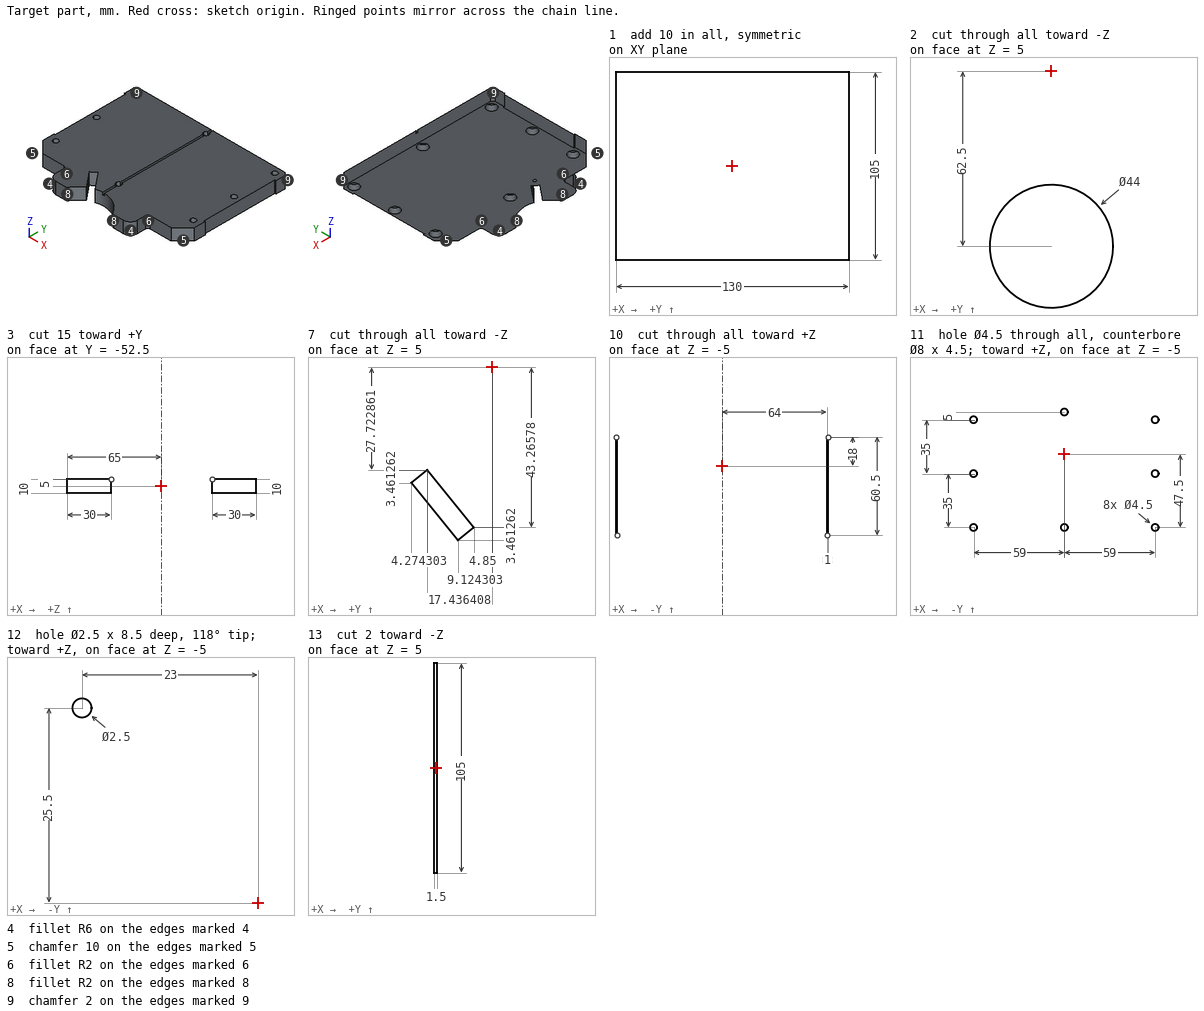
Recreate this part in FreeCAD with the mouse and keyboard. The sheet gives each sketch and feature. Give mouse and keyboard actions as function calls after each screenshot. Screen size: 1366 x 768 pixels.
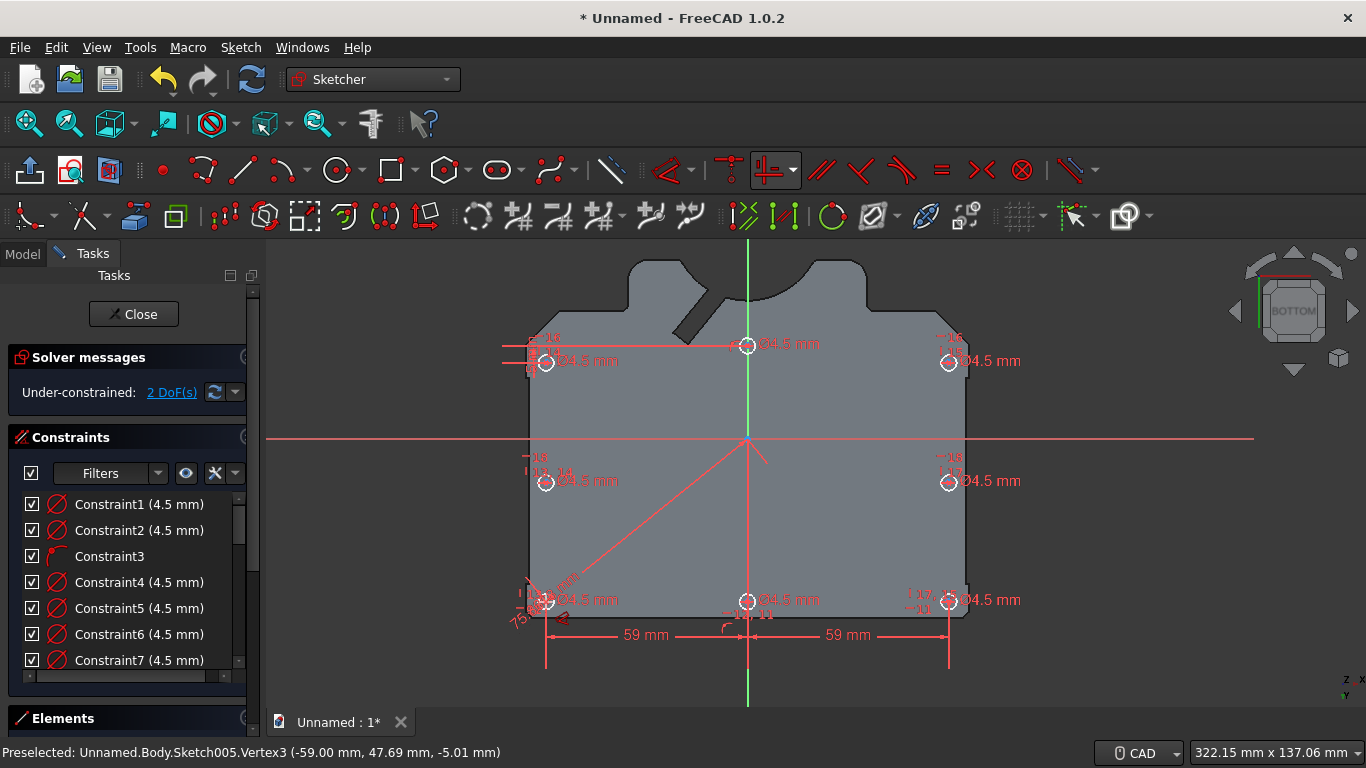
click(546, 483)
click(512, 542)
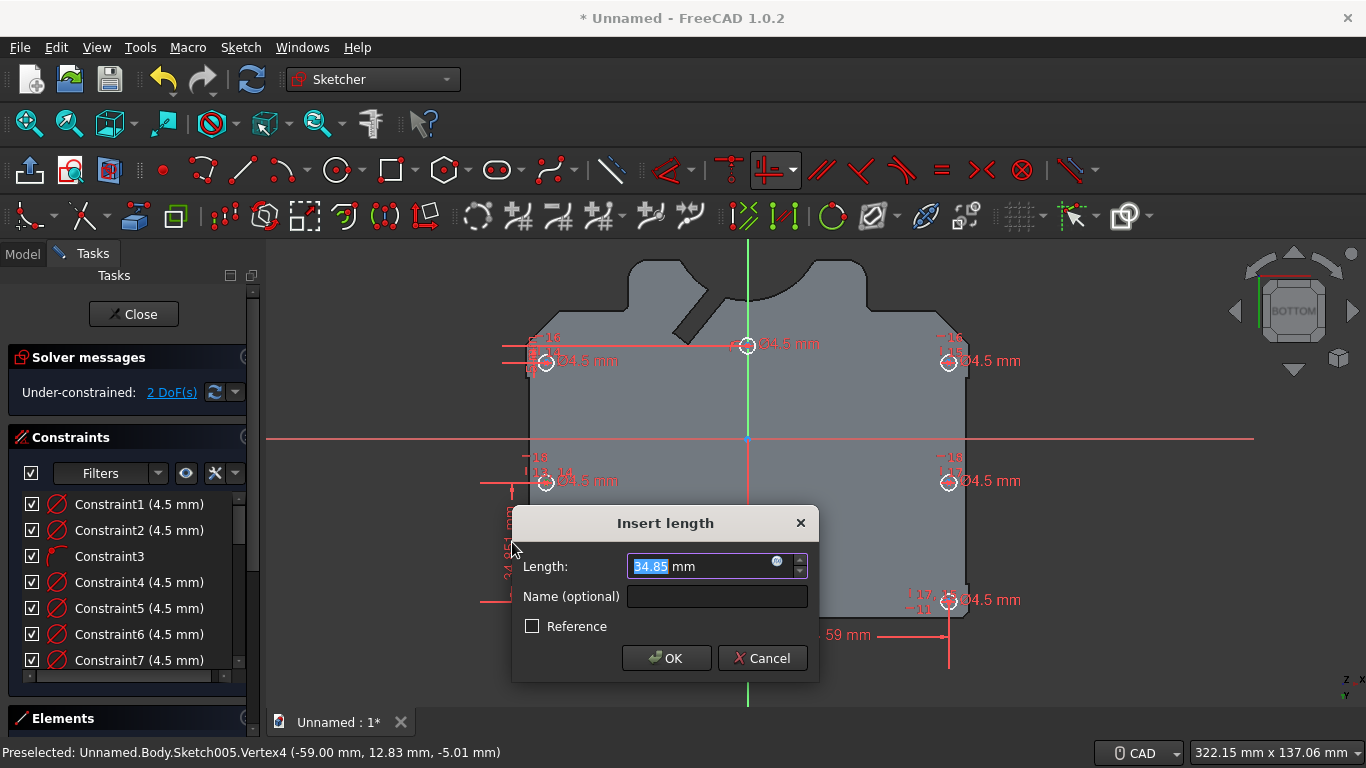
text(35)
key(Return)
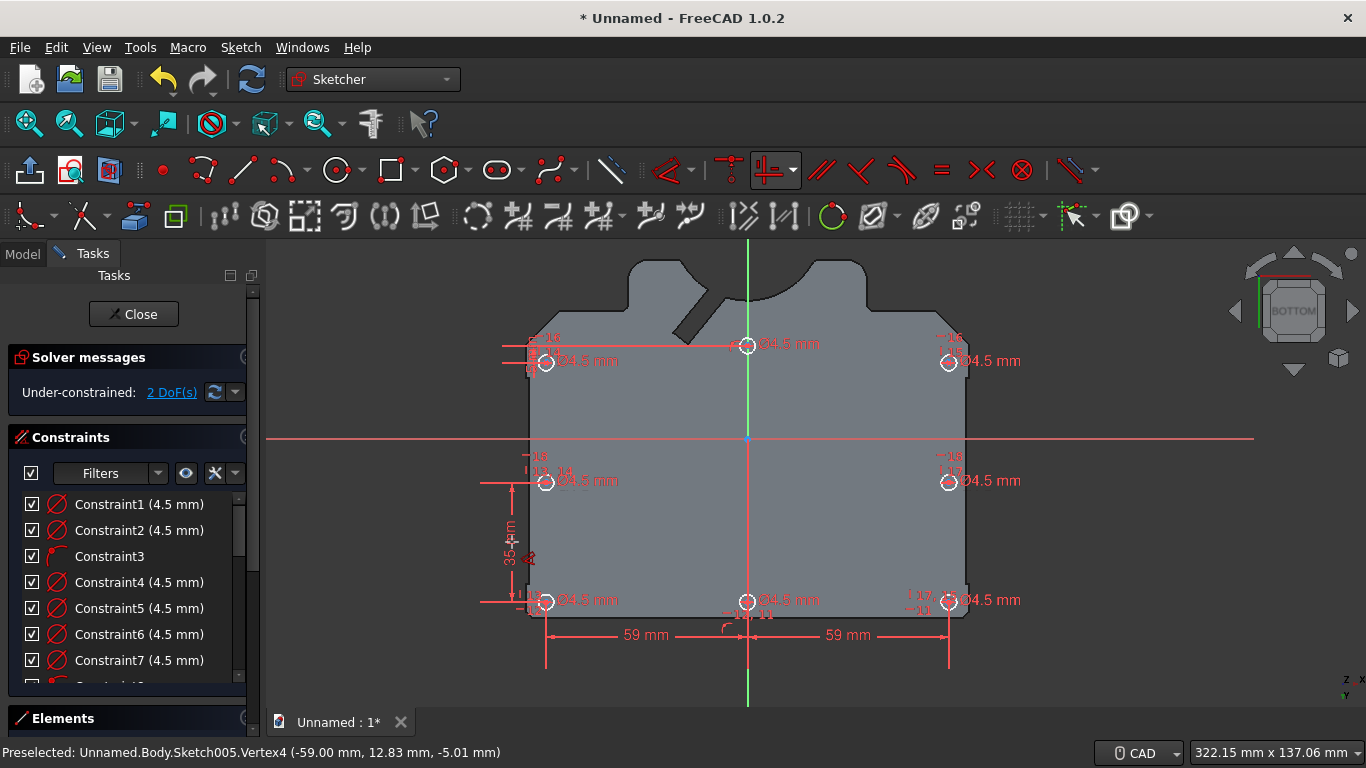
click(546, 483)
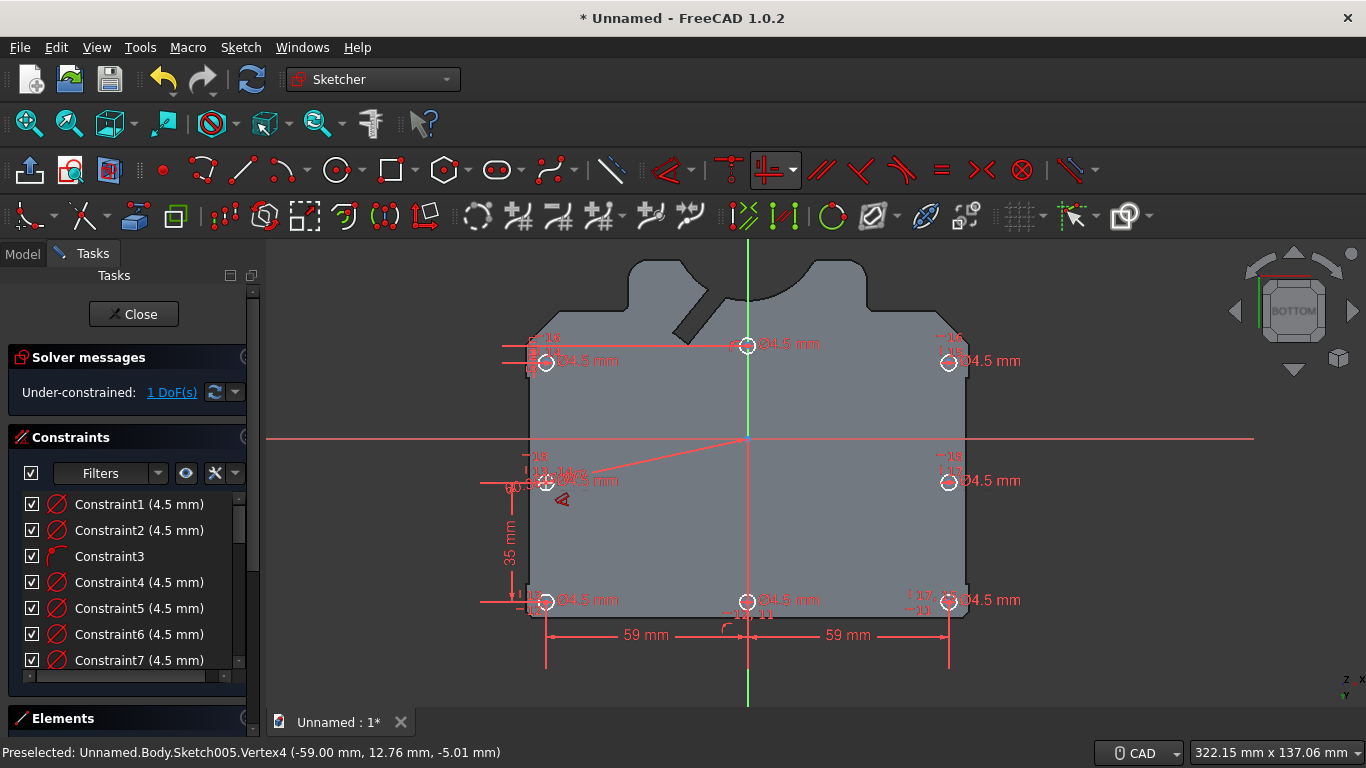
click(546, 363)
click(512, 423)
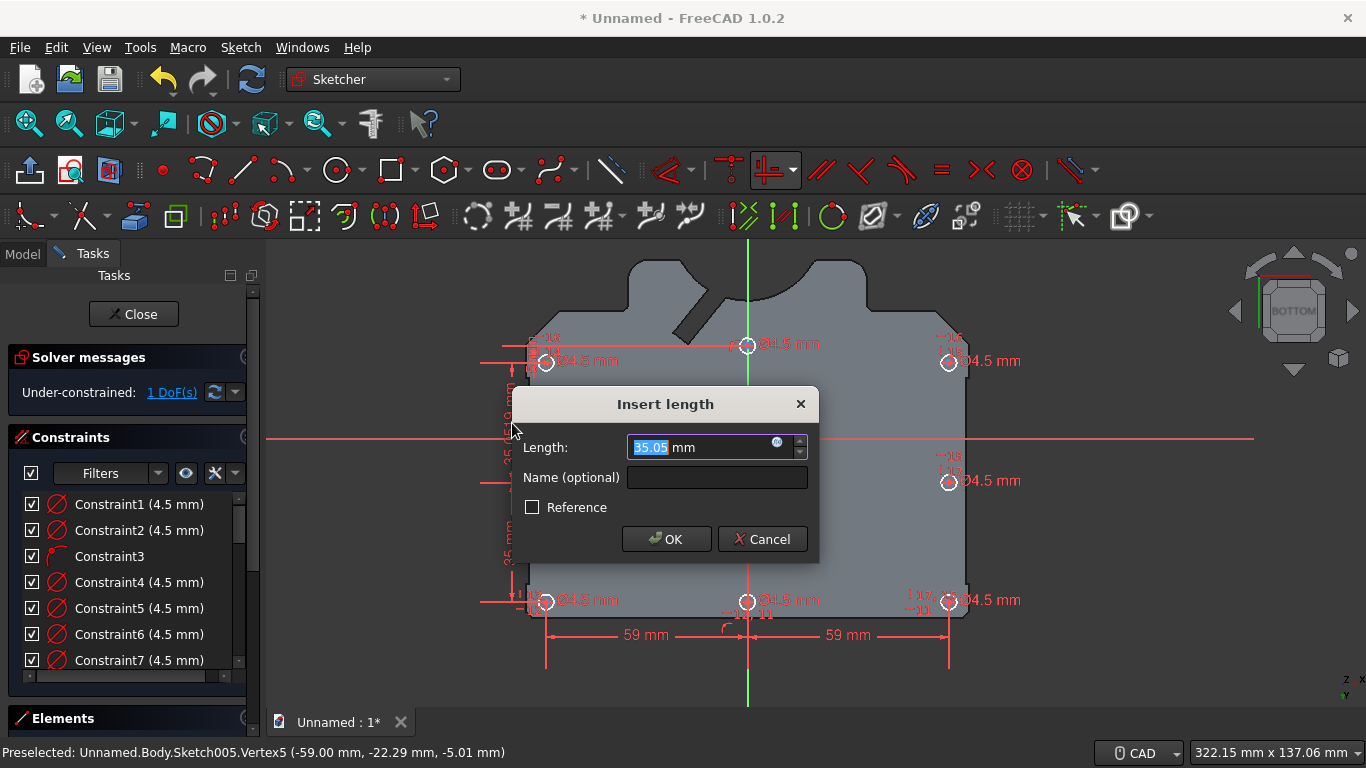
text(35)
key(Return)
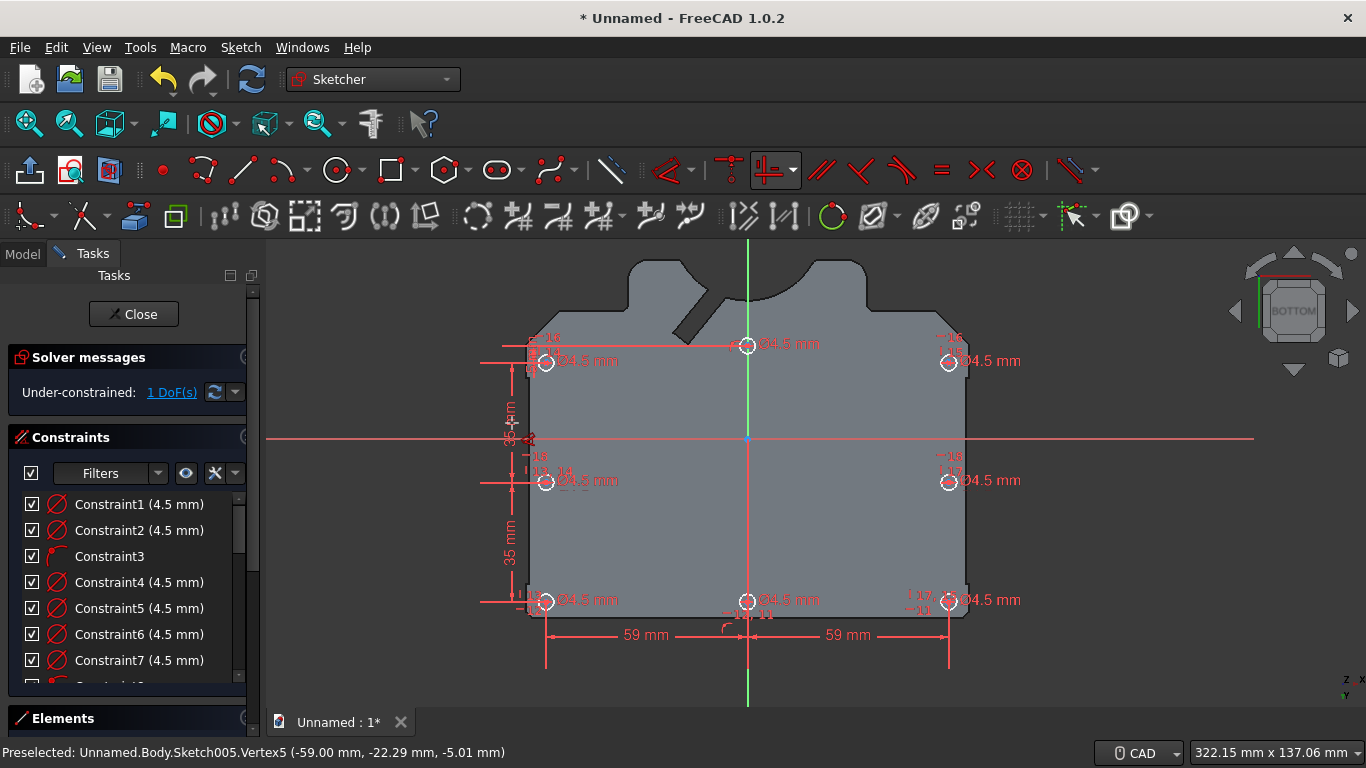
click(949, 602)
click(983, 521)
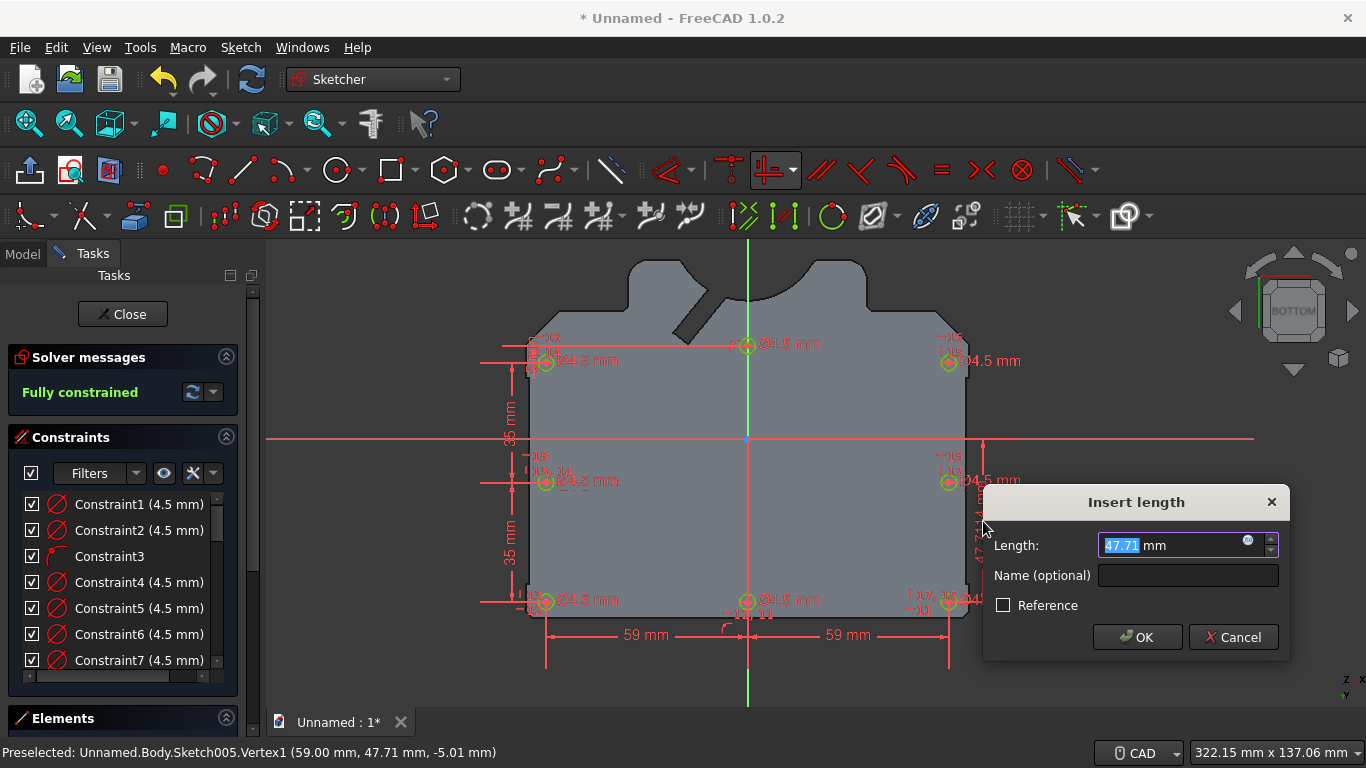
text(47.5)
key(Return)
key(Escape)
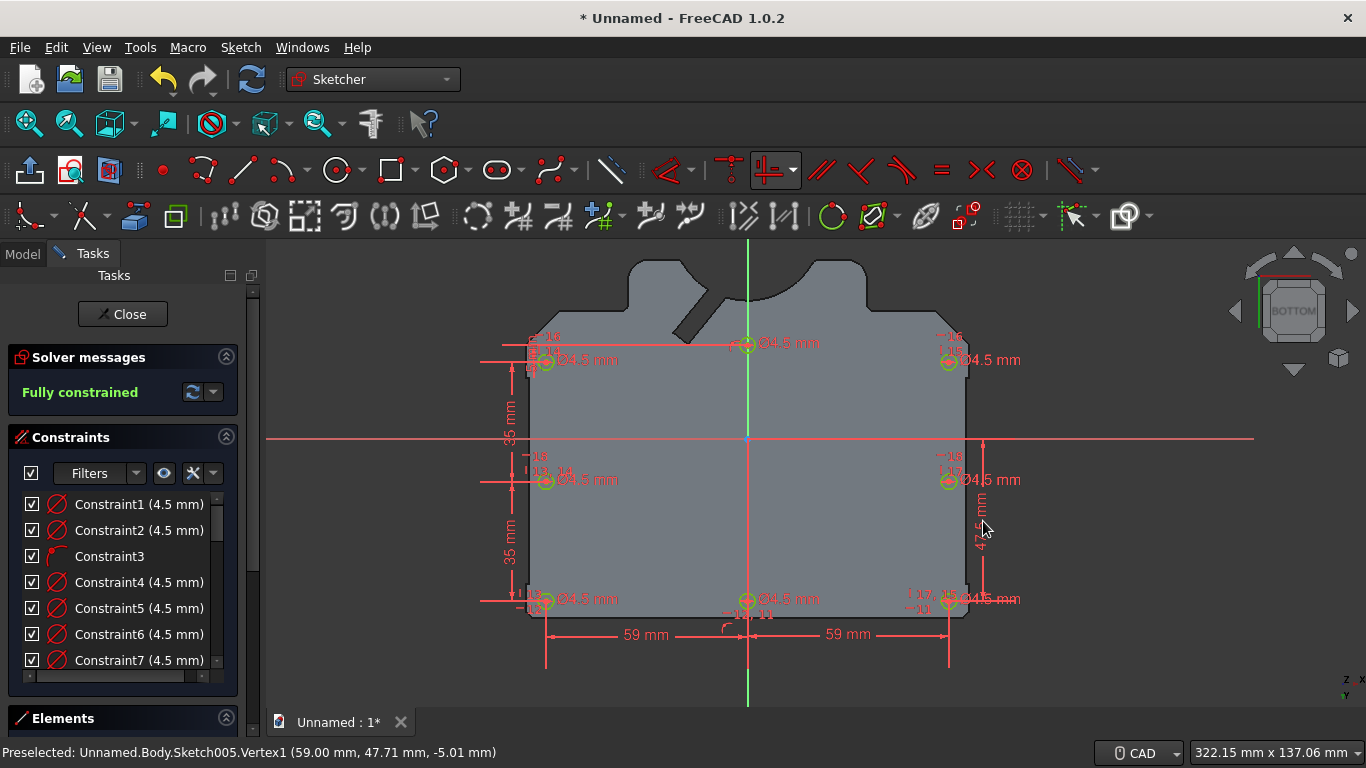
click(123, 314)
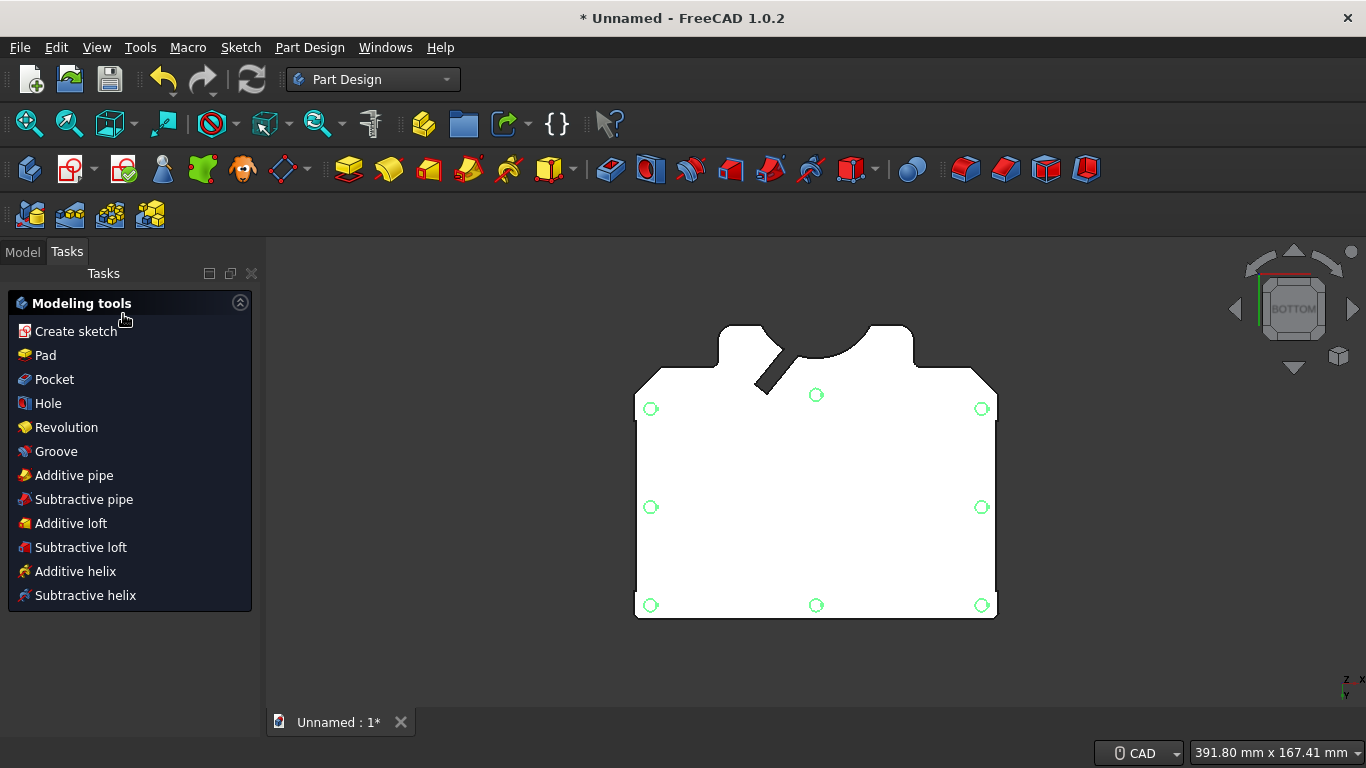
click(652, 170)